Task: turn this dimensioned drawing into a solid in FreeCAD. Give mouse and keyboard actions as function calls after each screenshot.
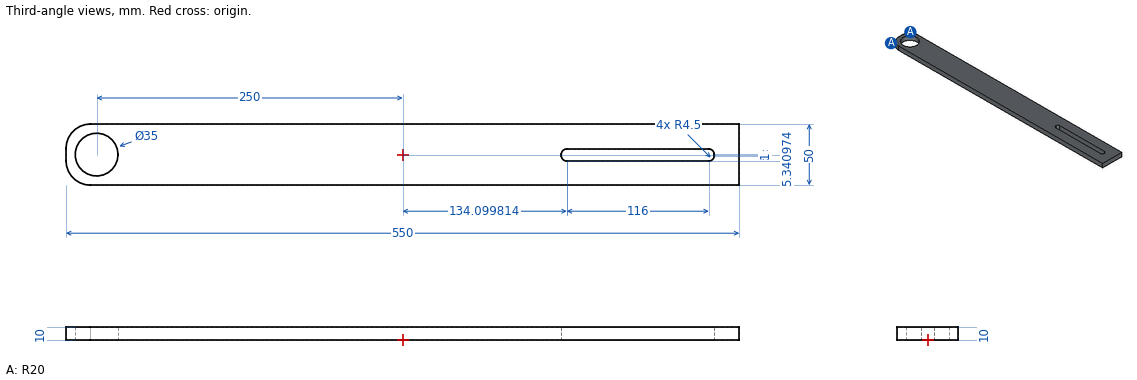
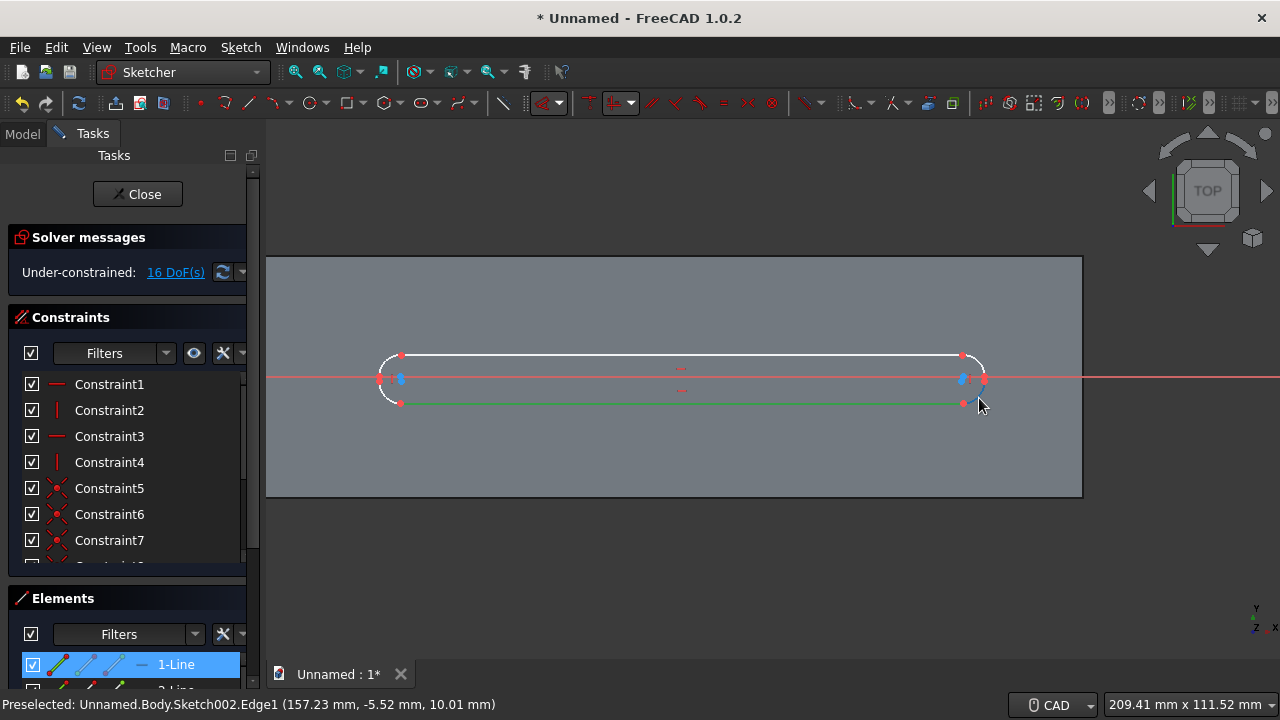
click(978, 397)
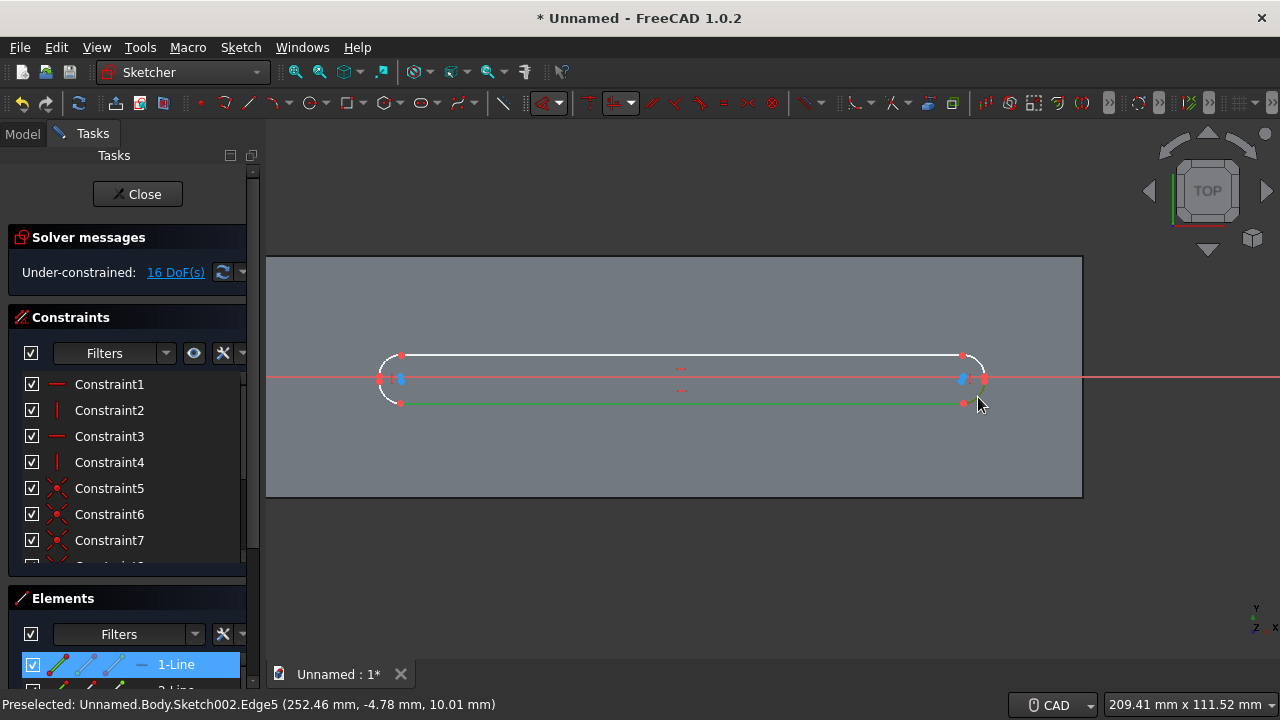
key(t)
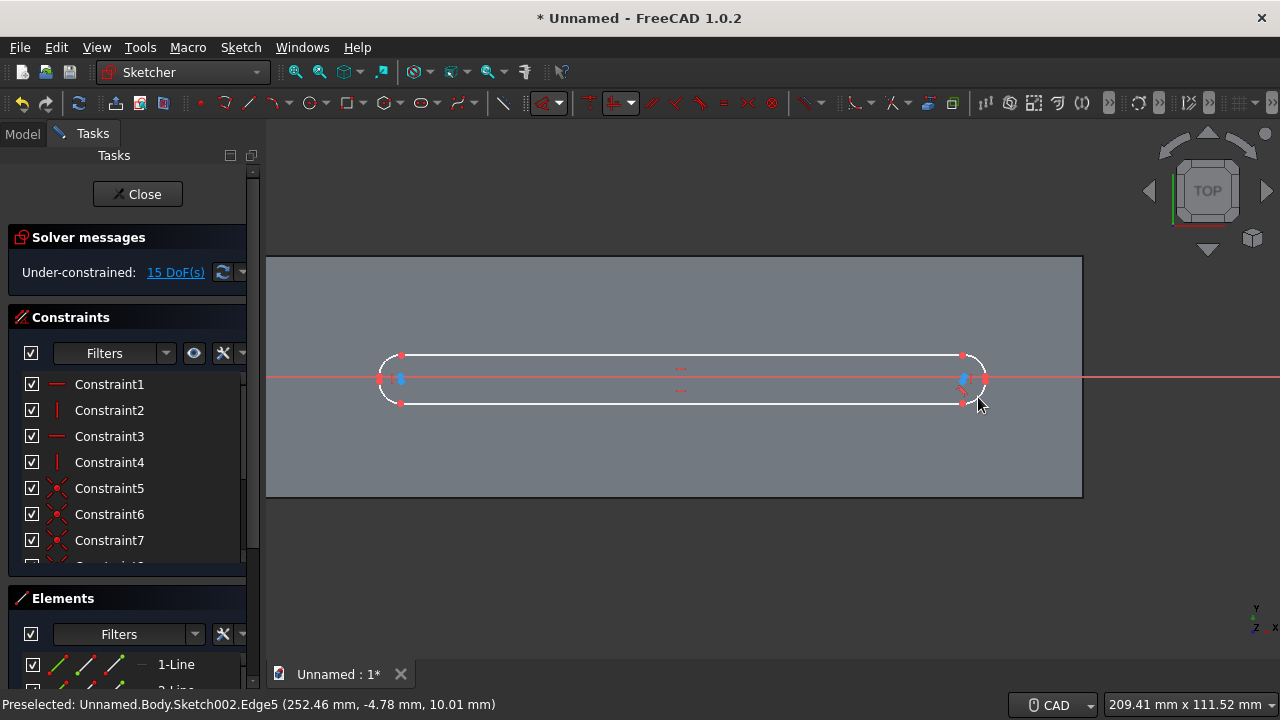
click(569, 404)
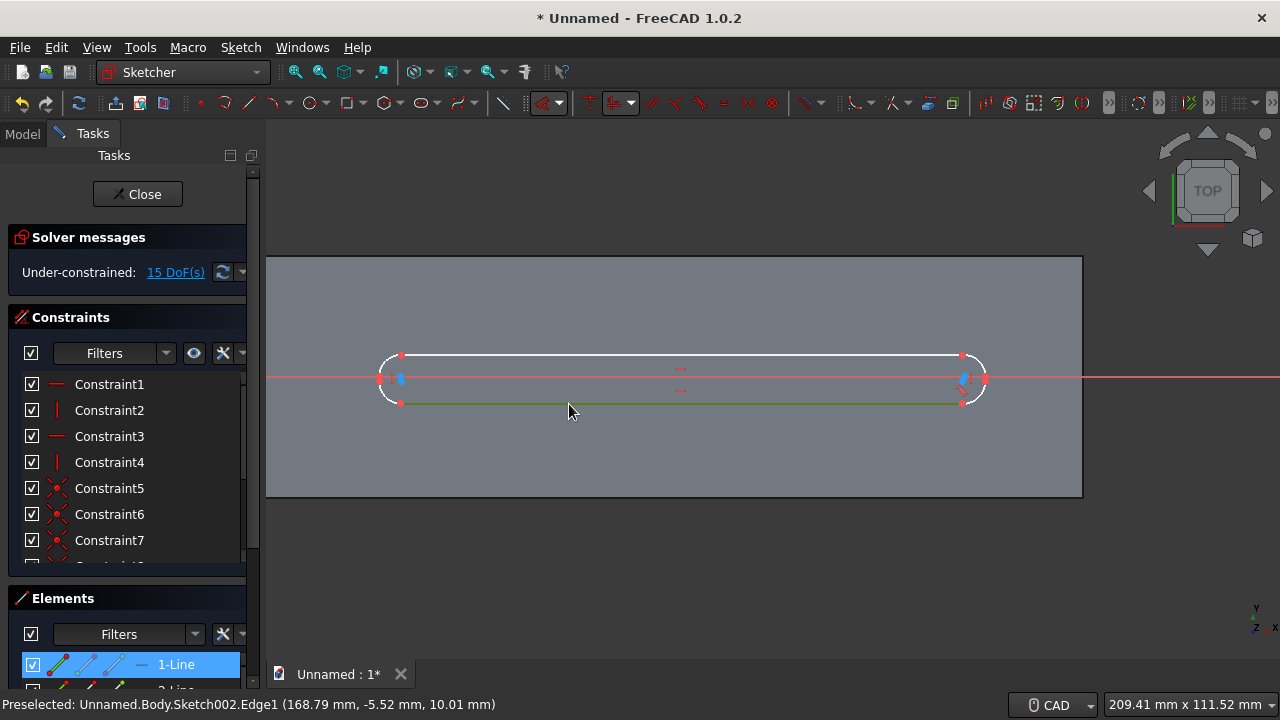
scroll(382, 391, up, 2)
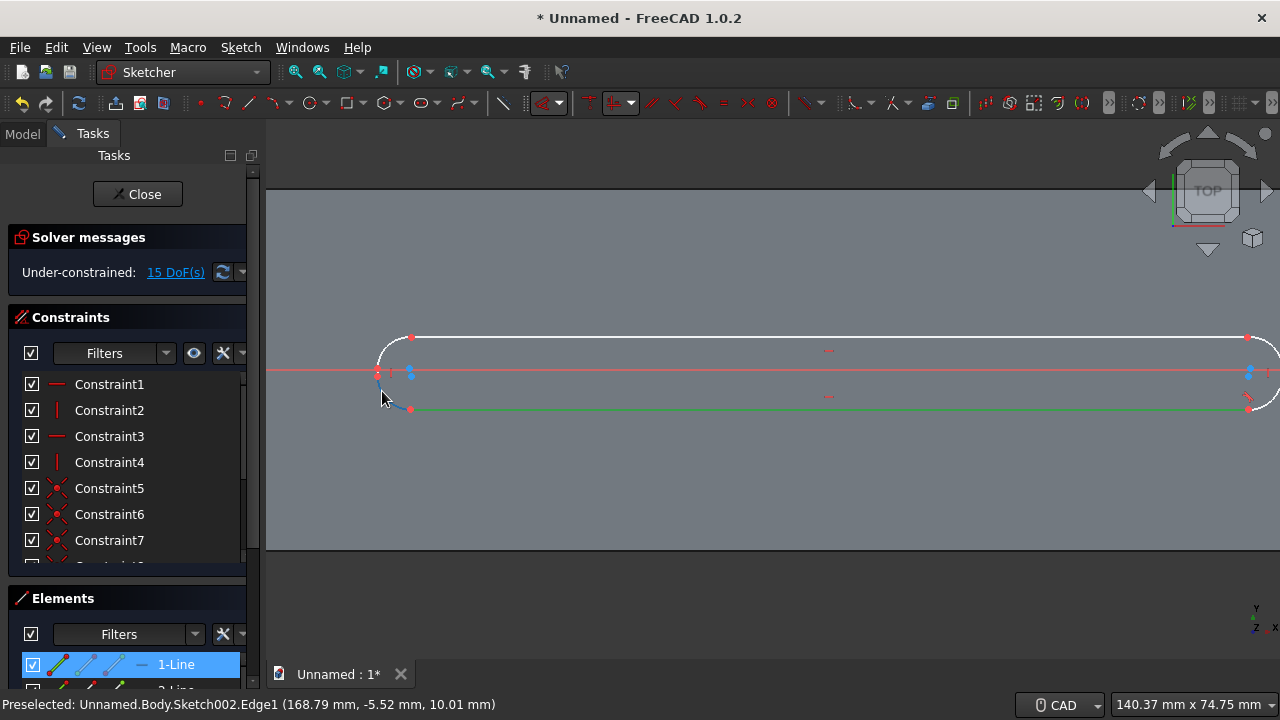
click(381, 391)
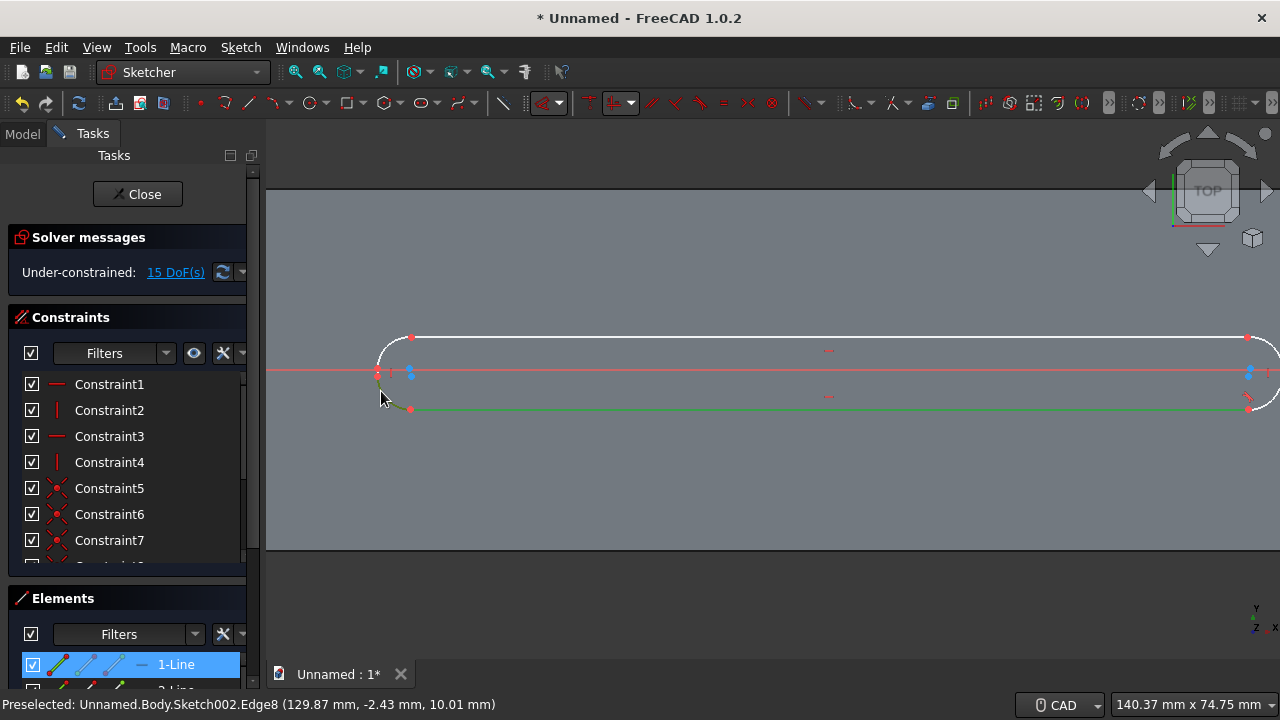
click(700, 104)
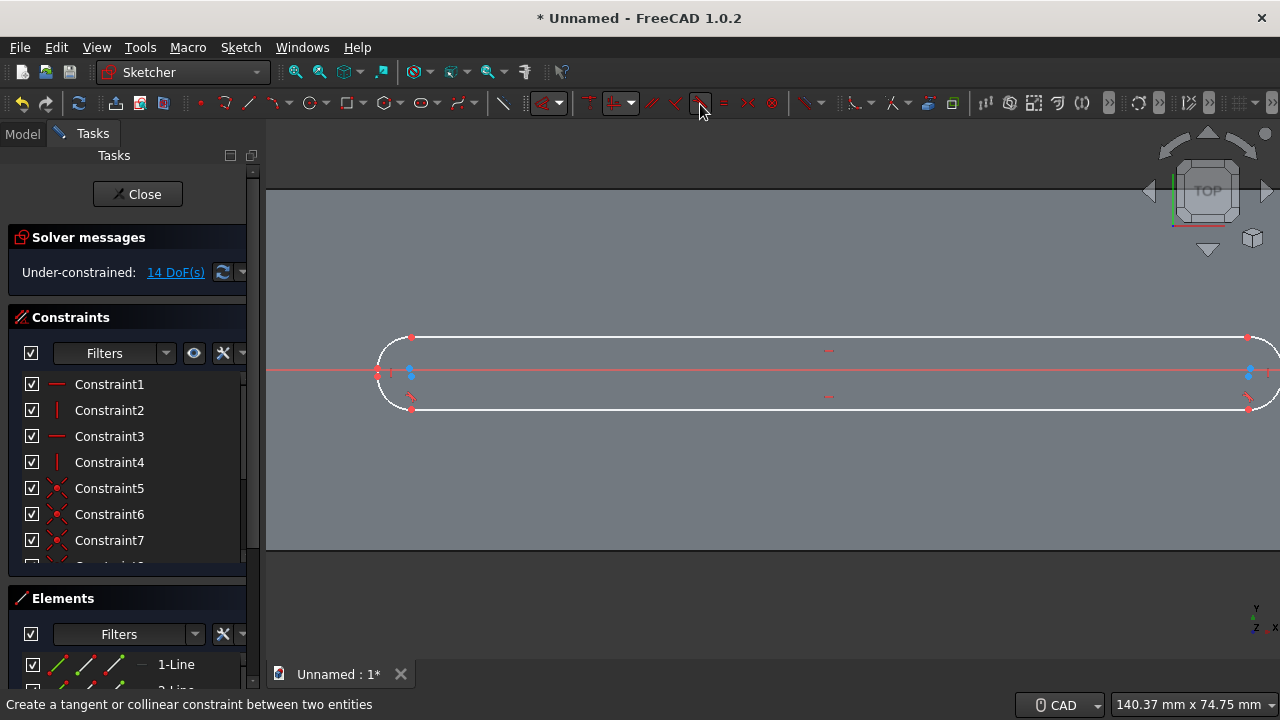
scroll(852, 396, down, 6)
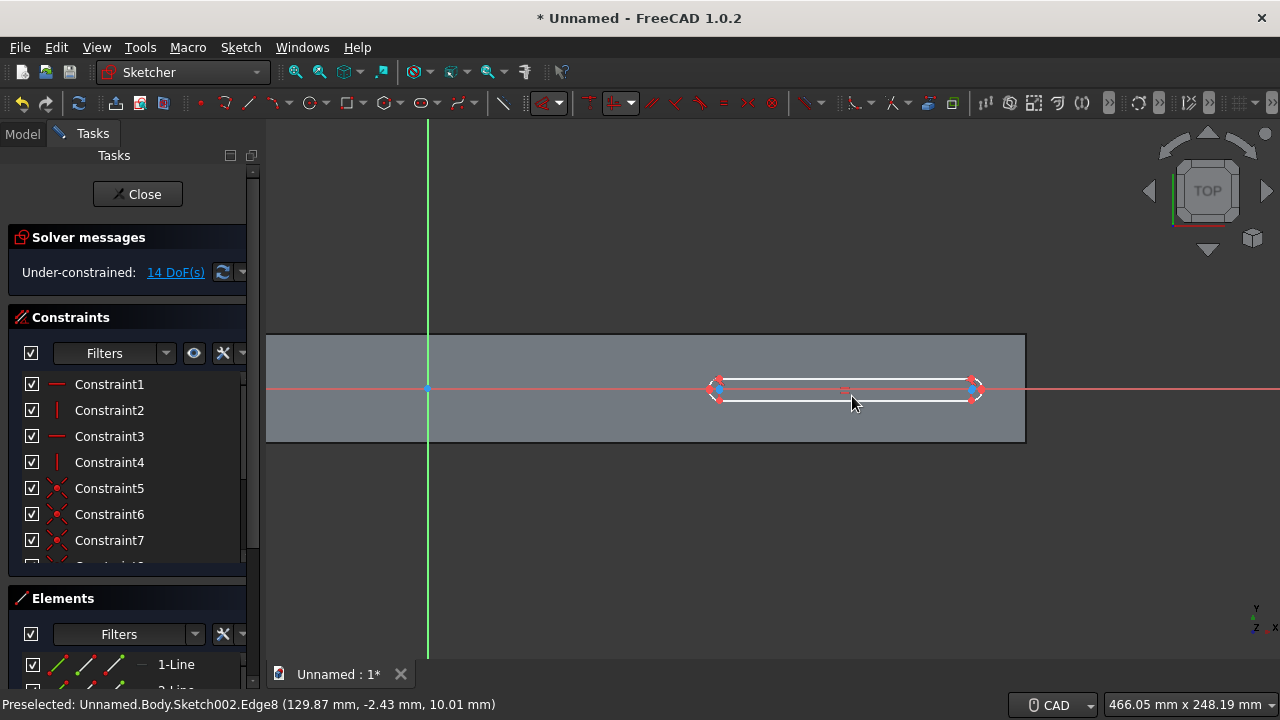
scroll(982, 389, up, 13)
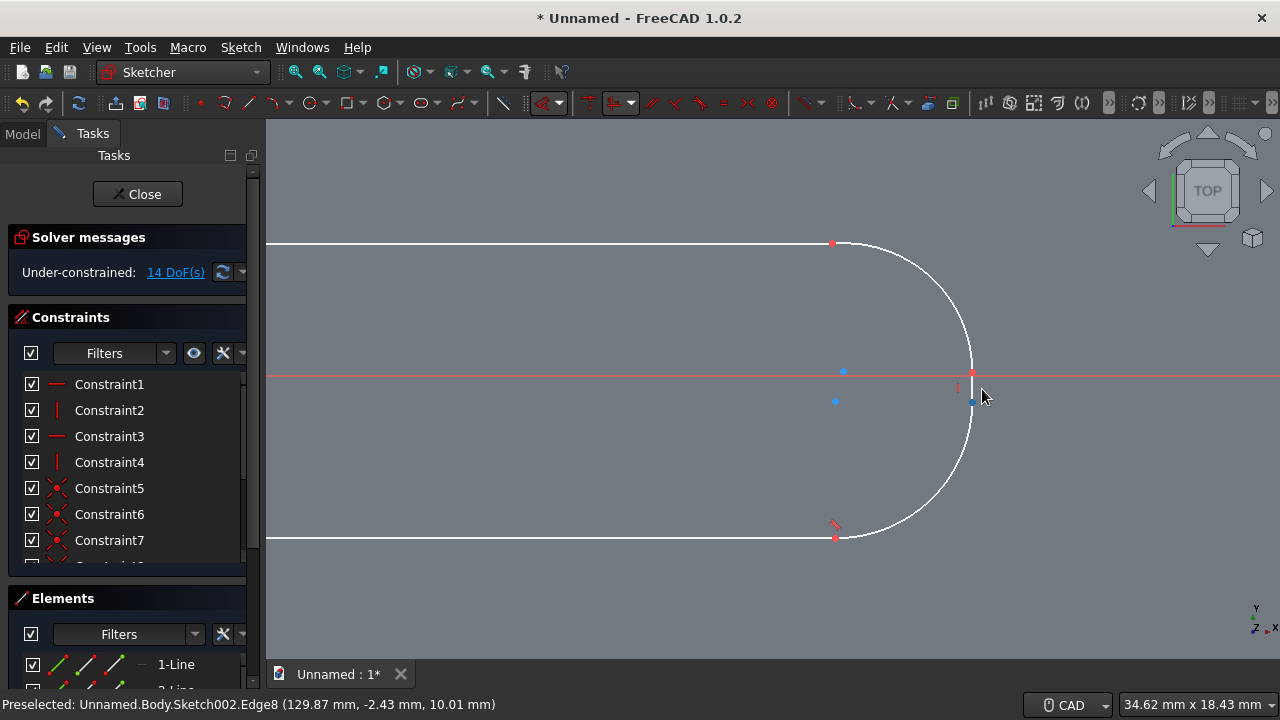
click(972, 387)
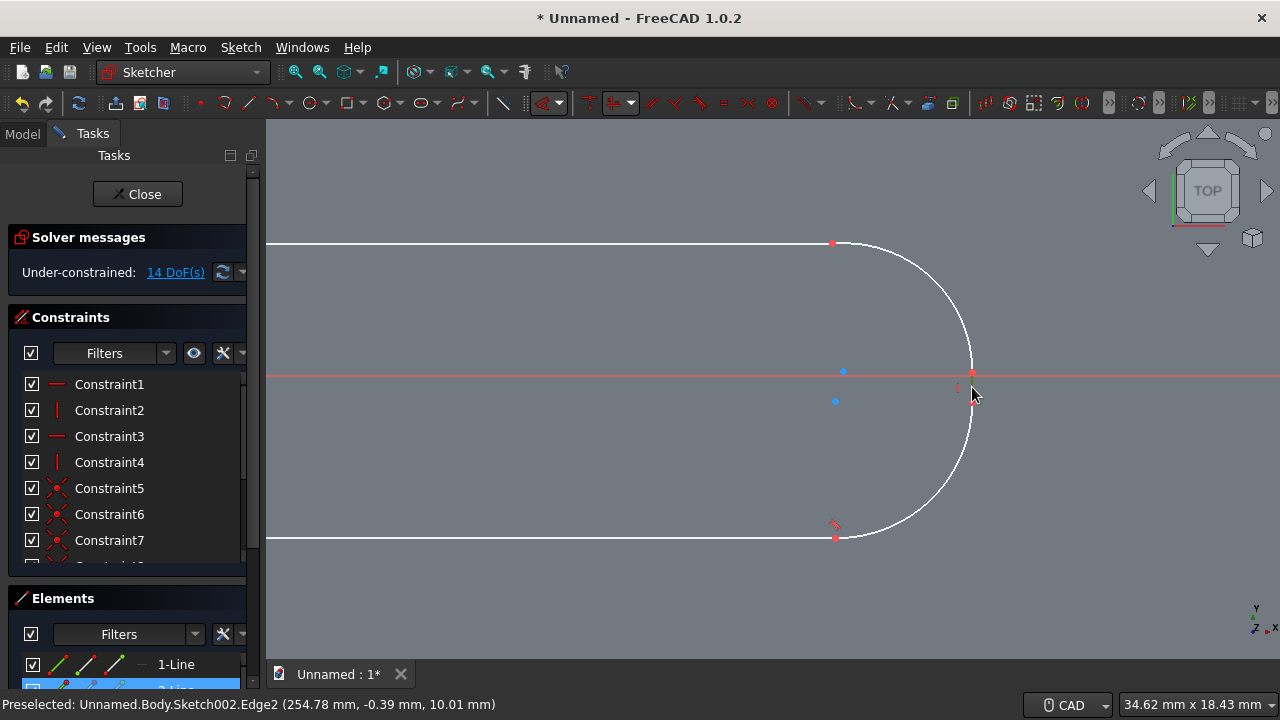
scroll(983, 389, down, 13)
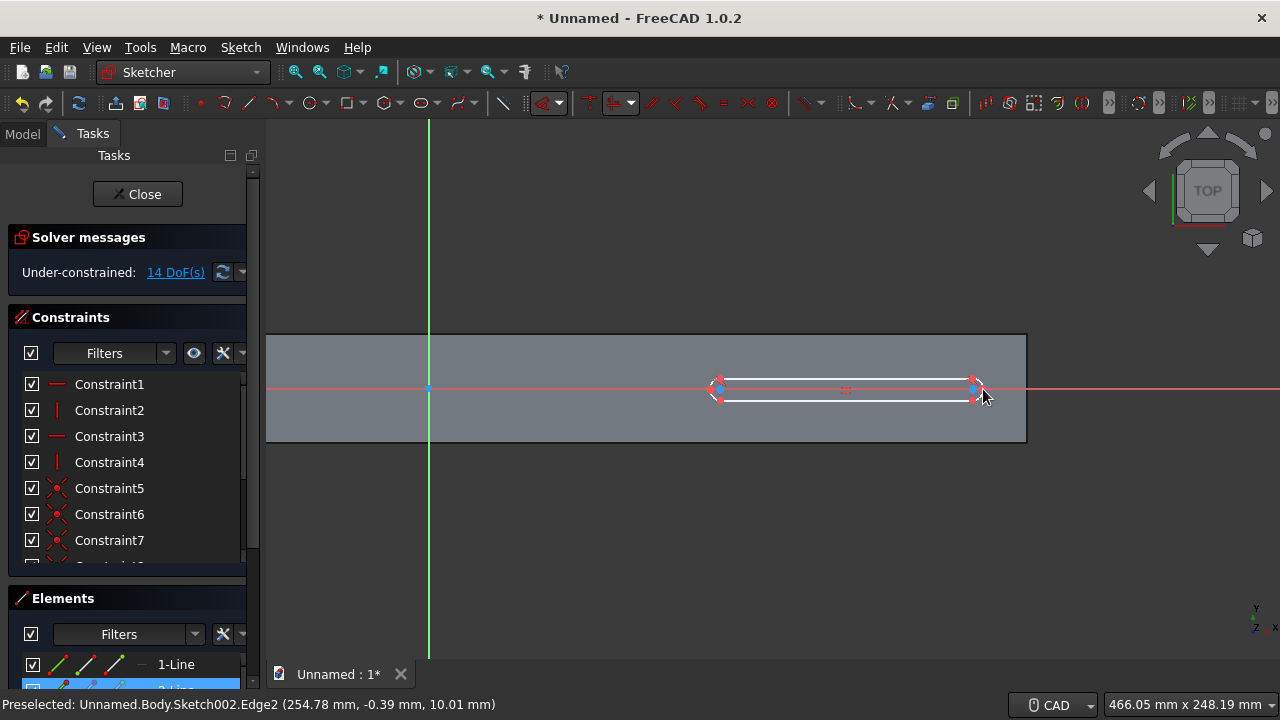
scroll(977, 399, up, 6)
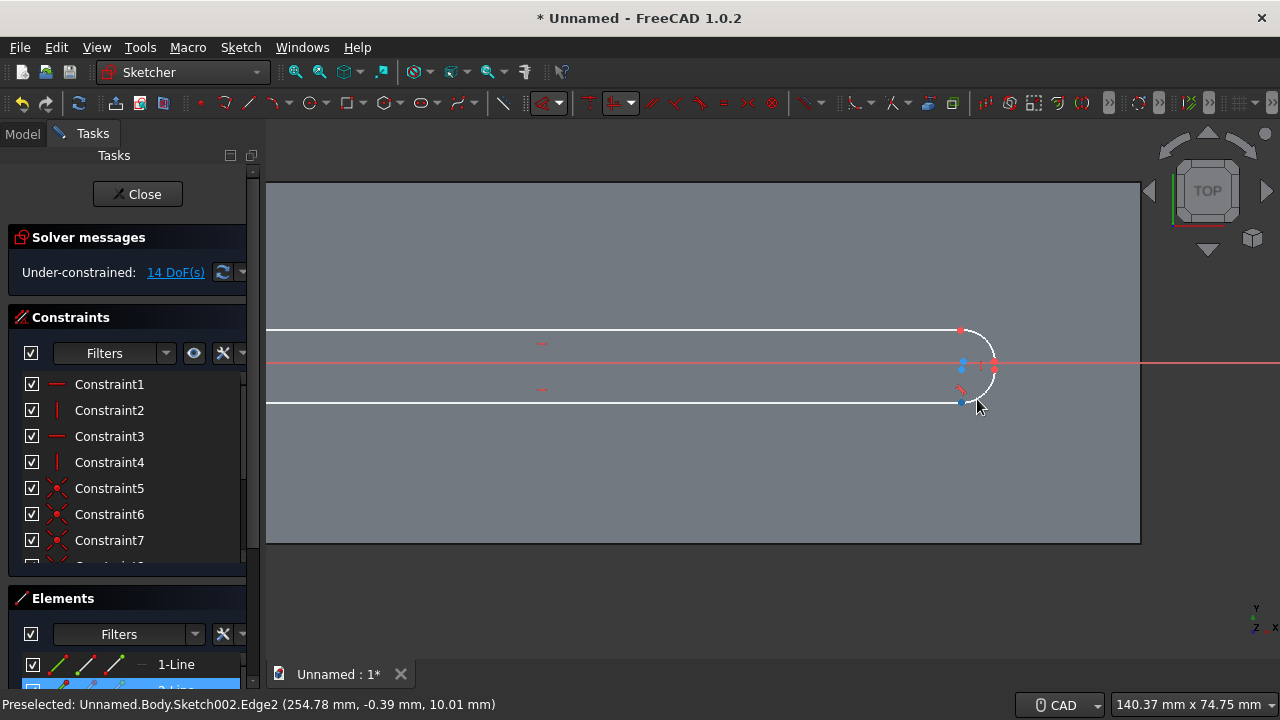
click(976, 399)